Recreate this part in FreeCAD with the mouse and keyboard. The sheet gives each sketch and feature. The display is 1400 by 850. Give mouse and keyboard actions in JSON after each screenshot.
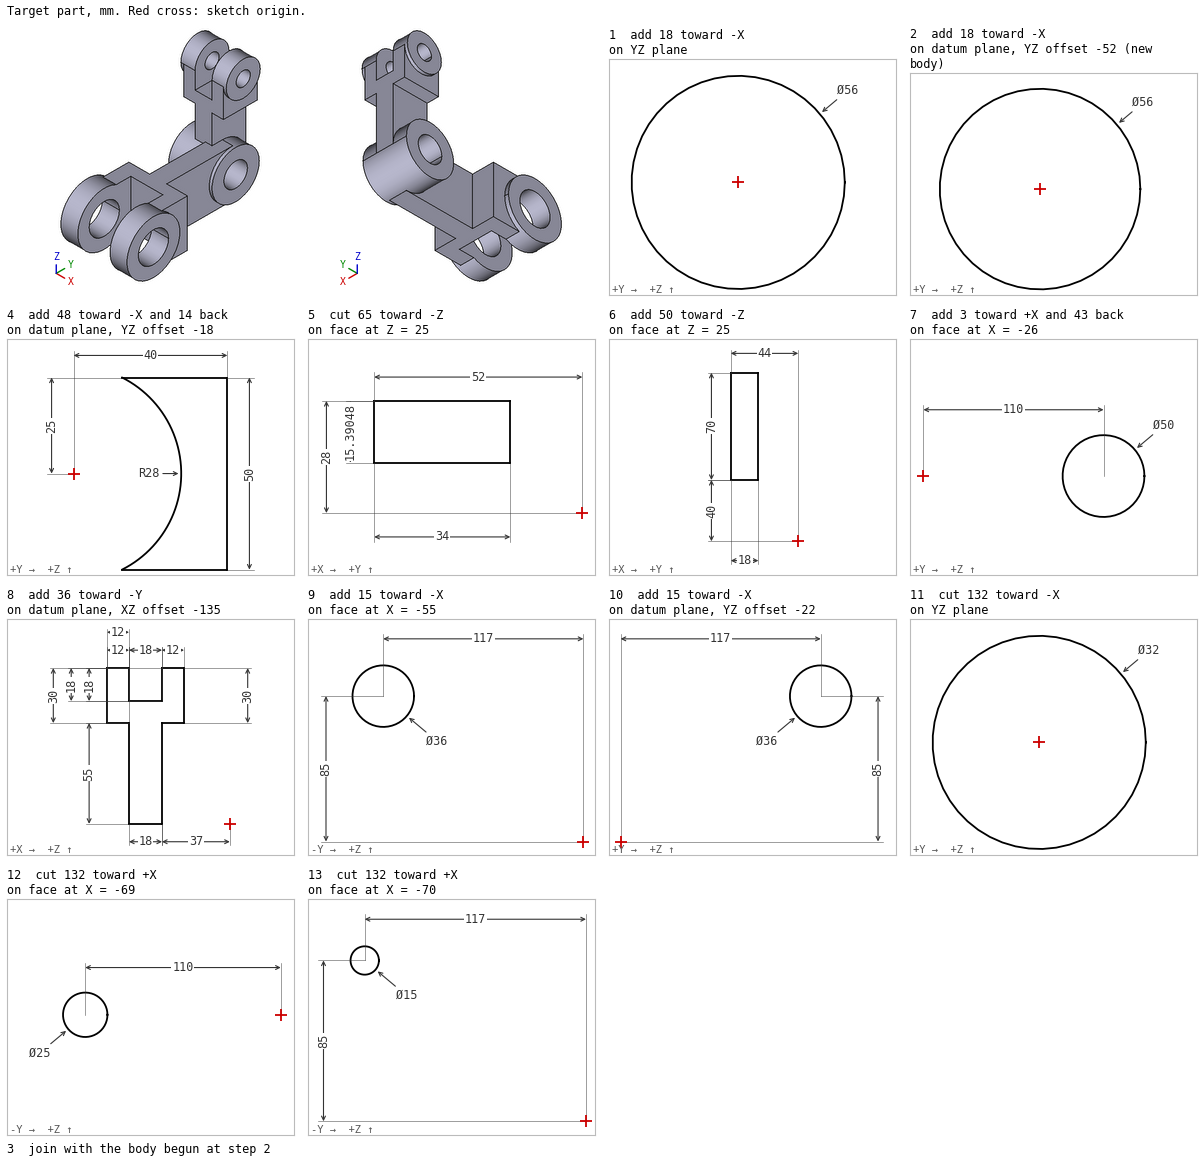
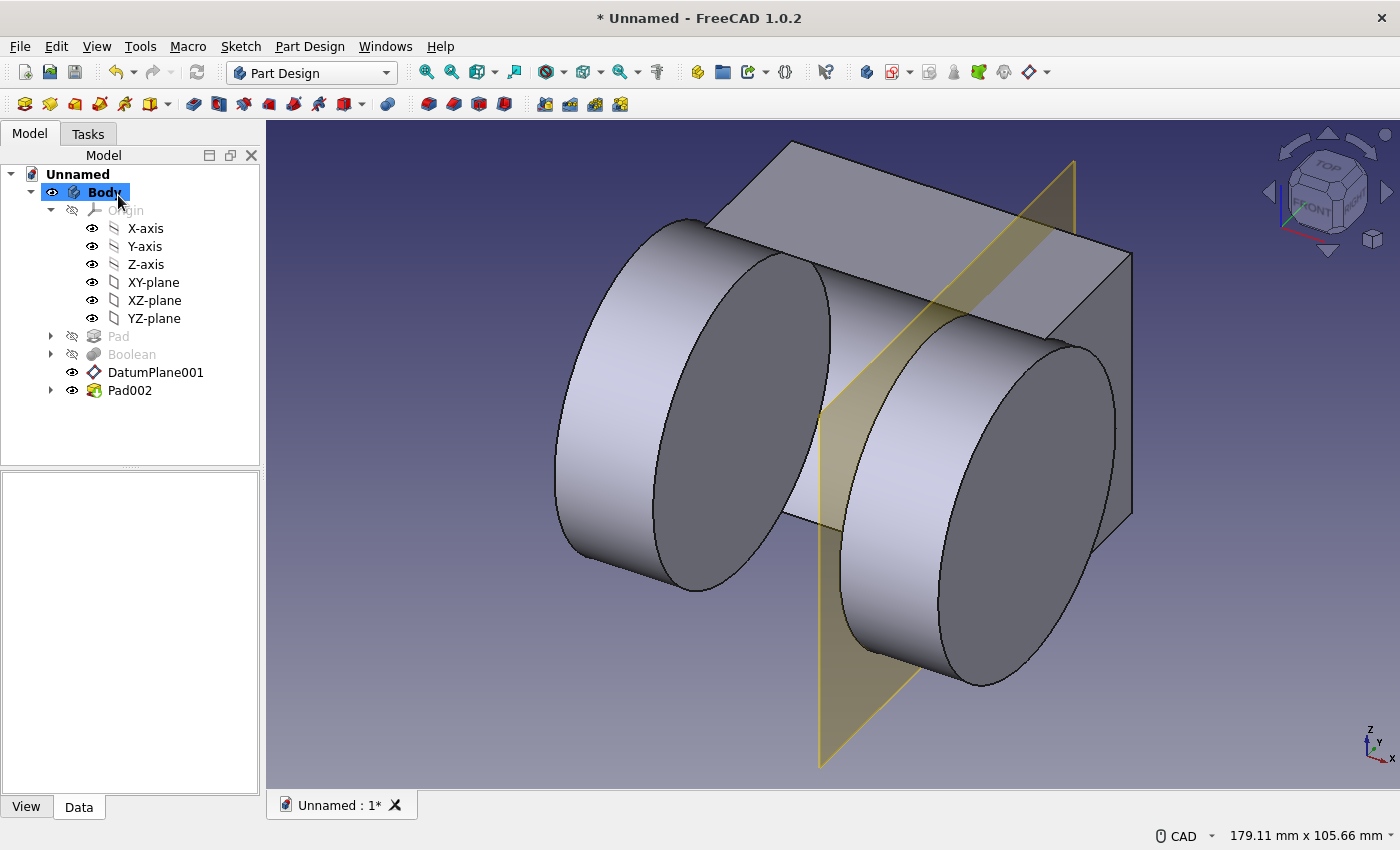
{"action": "left_click", "coordinate": [117, 372]}
{"action": "key", "text": "space"}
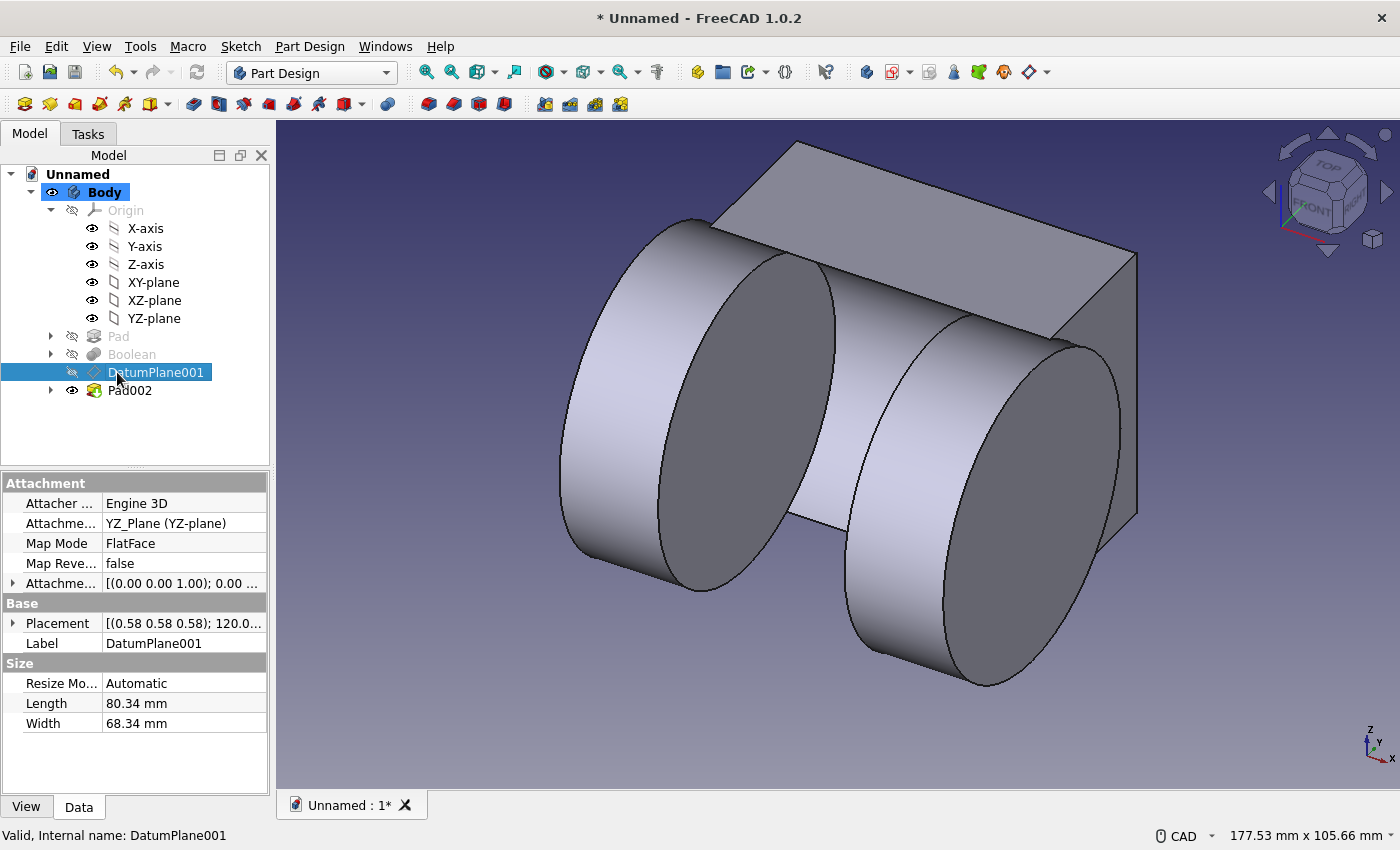
{"action": "key", "text": "v f"}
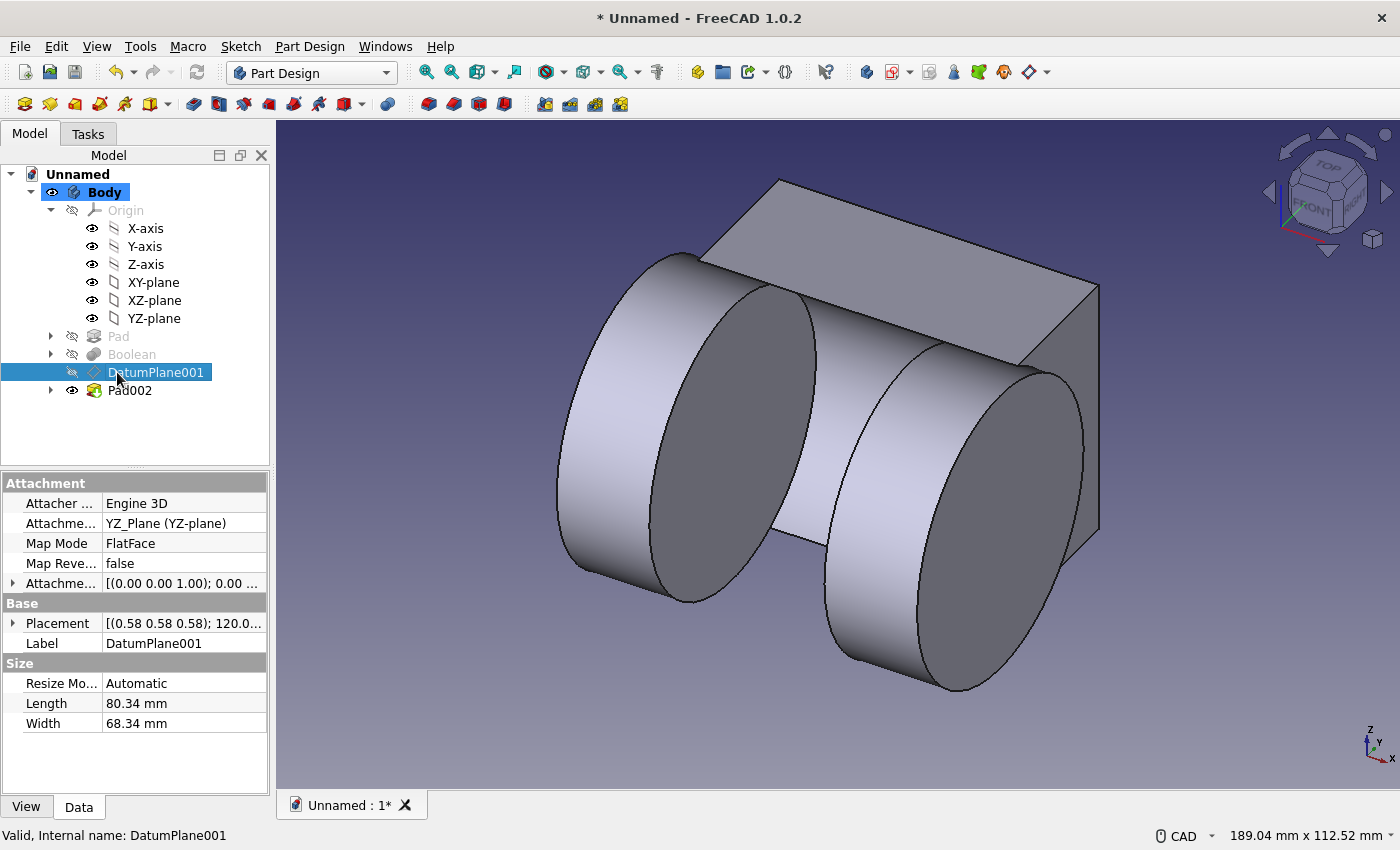
{"action": "left_click", "coordinate": [944, 287]}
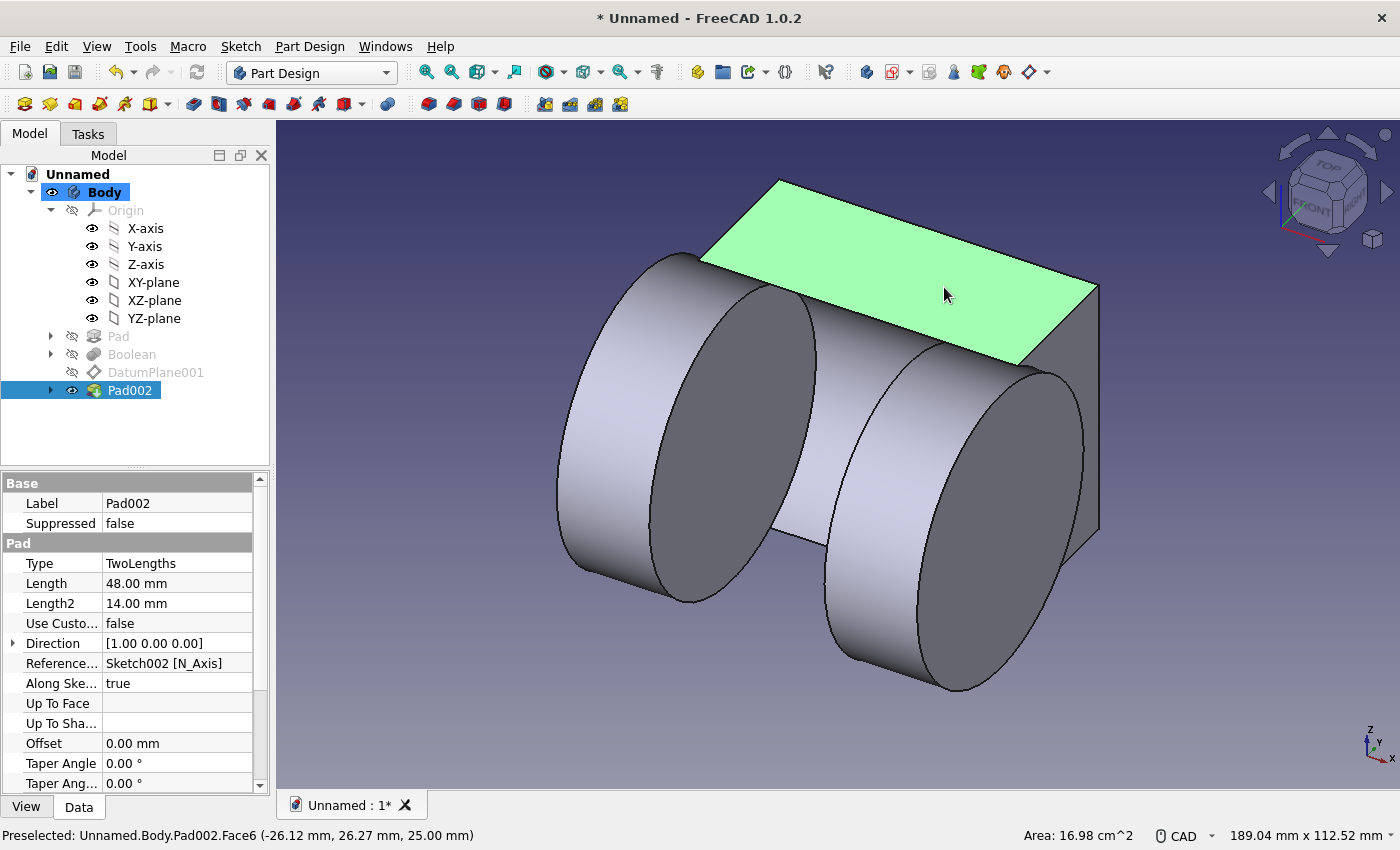
{"action": "left_click", "coordinate": [892, 72]}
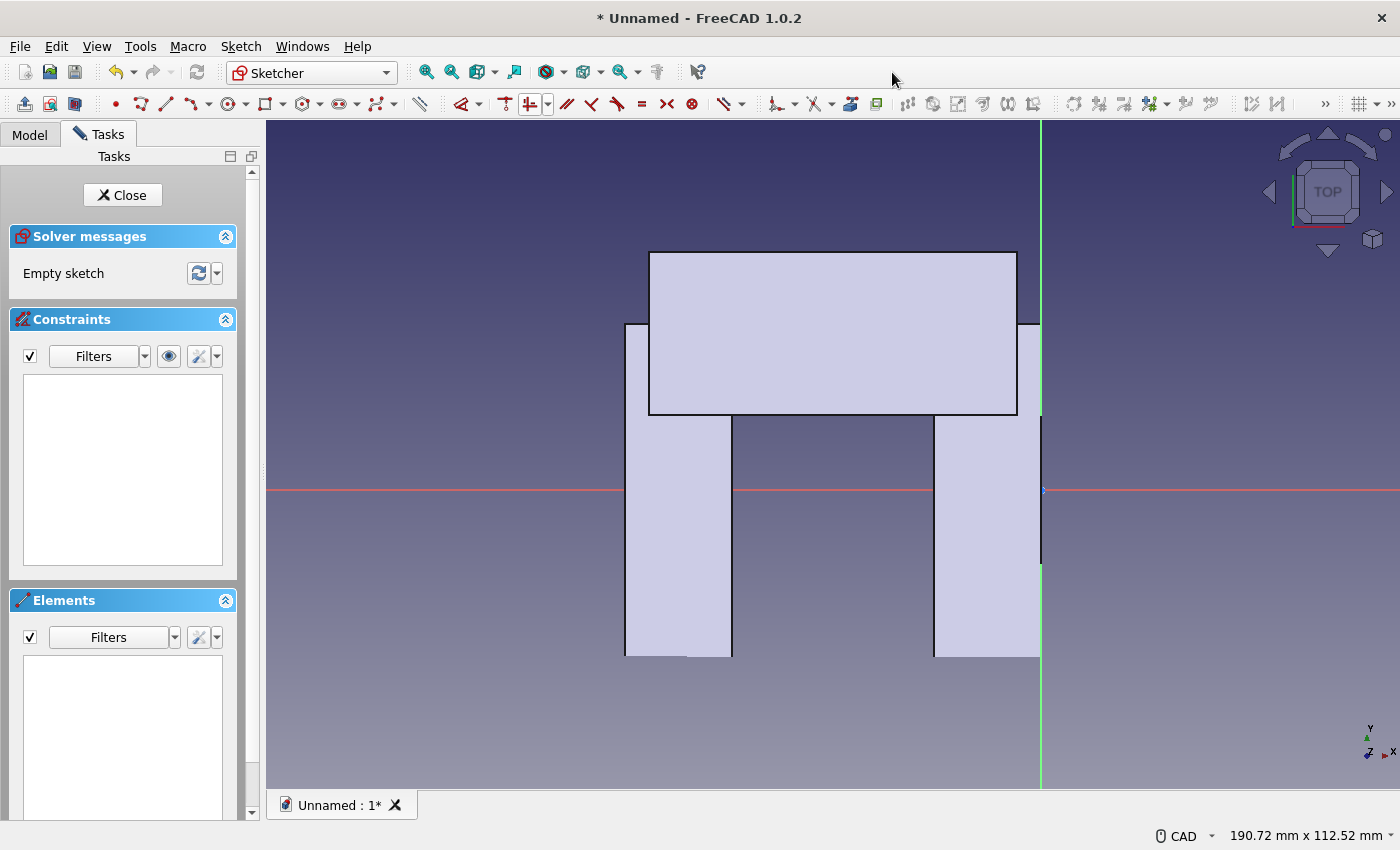
{"action": "left_click", "coordinate": [75, 104]}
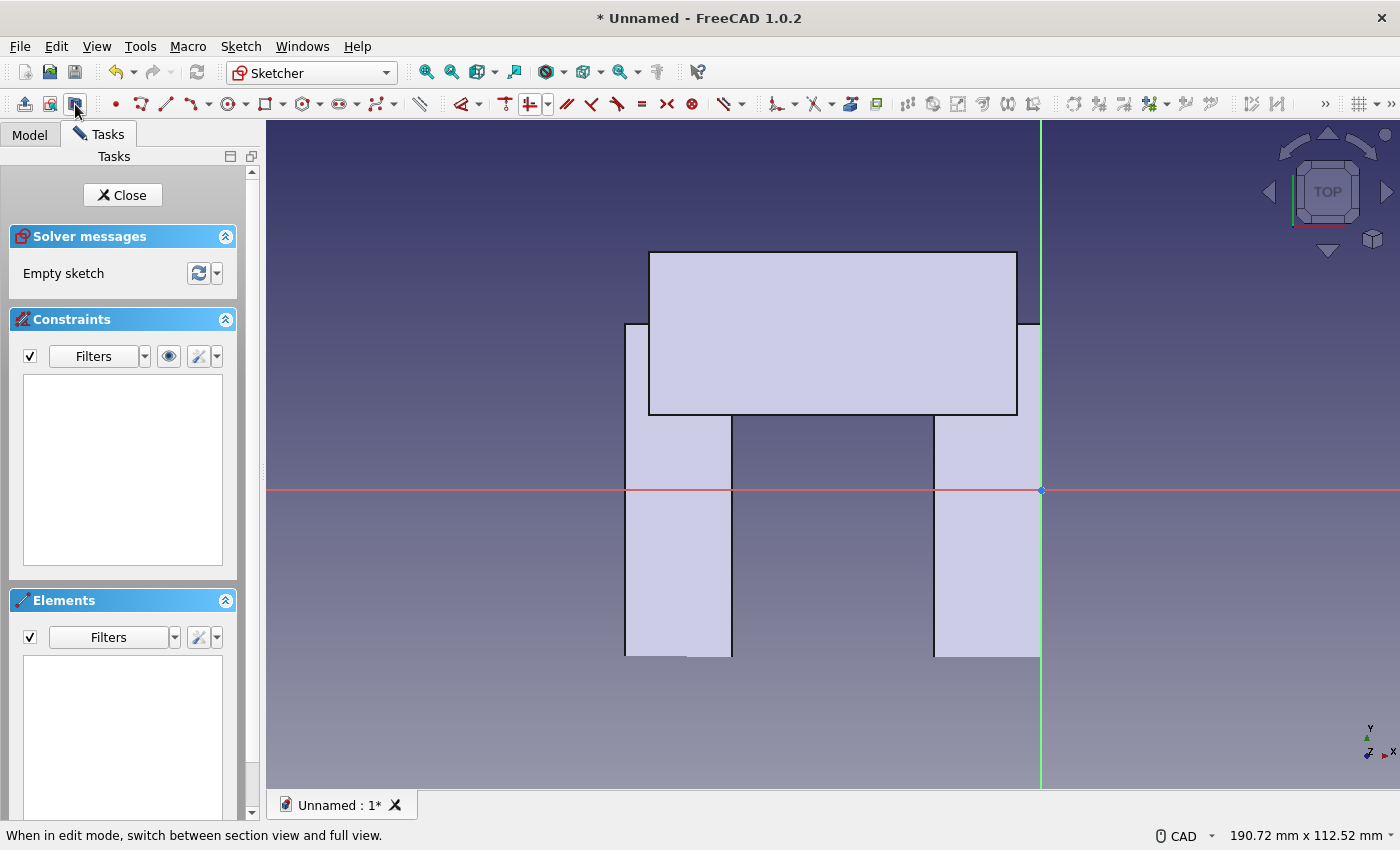
{"action": "scroll", "coordinate": [986, 368], "scroll_direction": "up", "scroll_amount": 4}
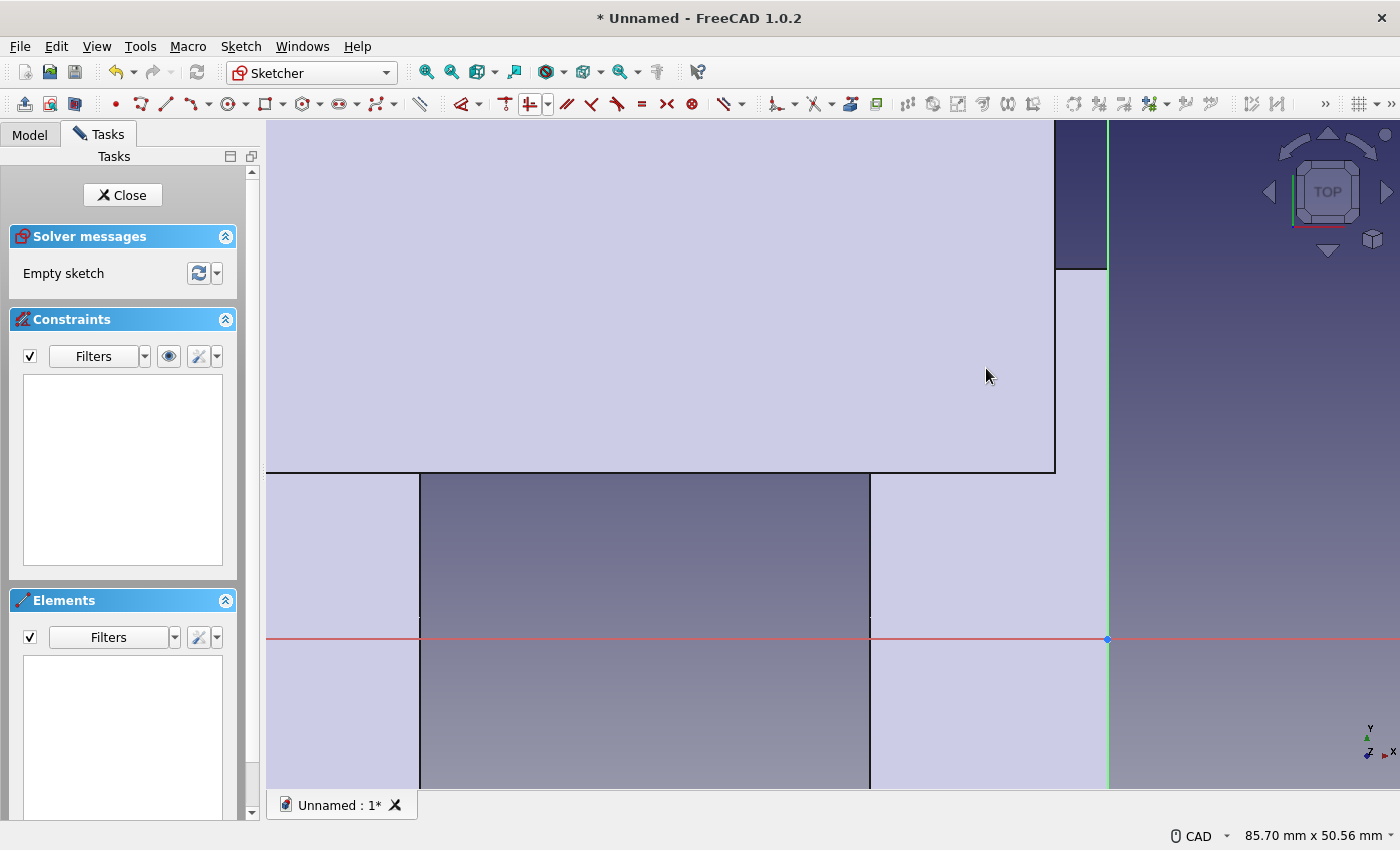
{"action": "key", "text": "g r"}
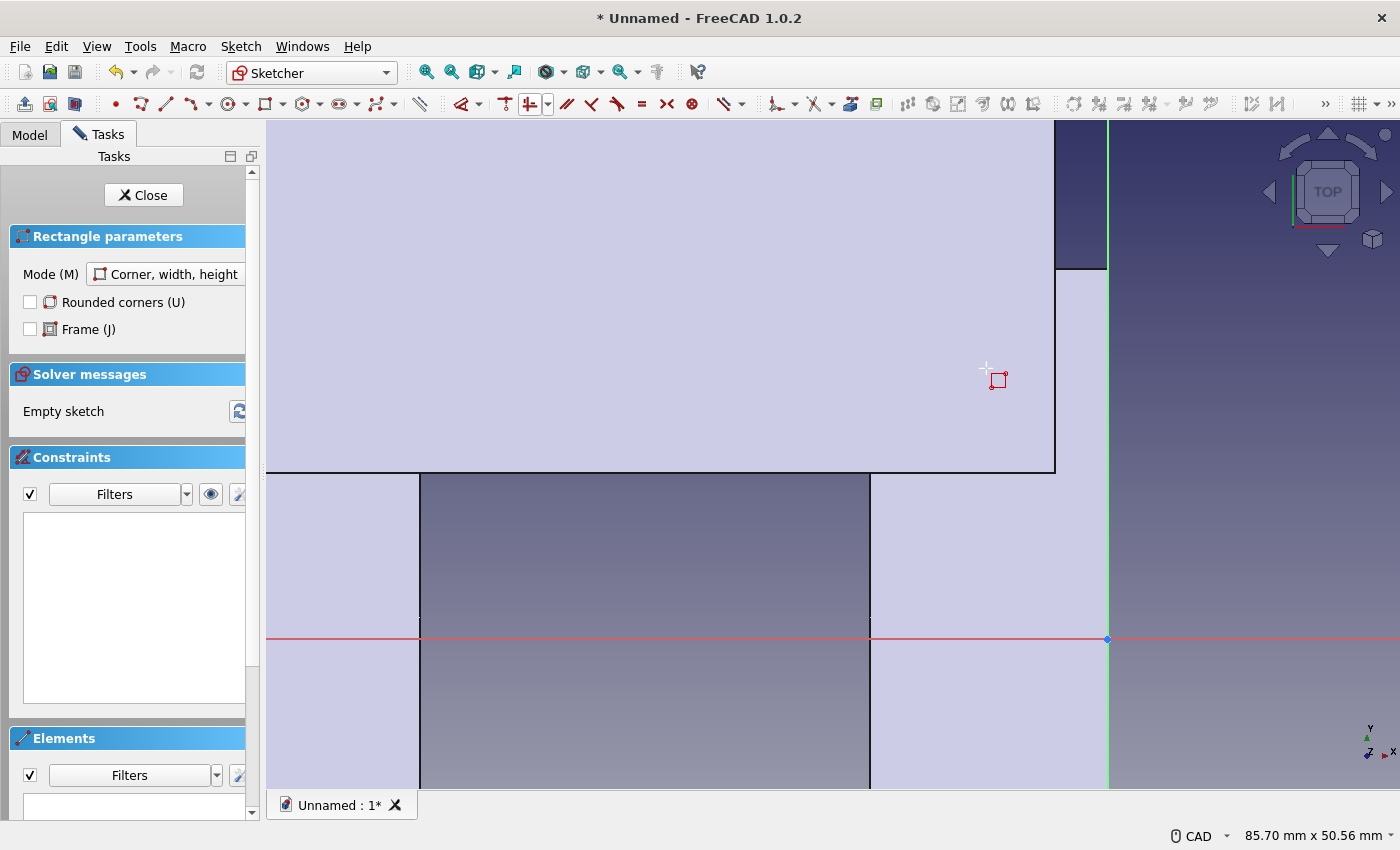
{"action": "left_click", "coordinate": [420, 269]}
{"action": "left_click", "coordinate": [870, 473]}
{"action": "key", "text": "Escape"}